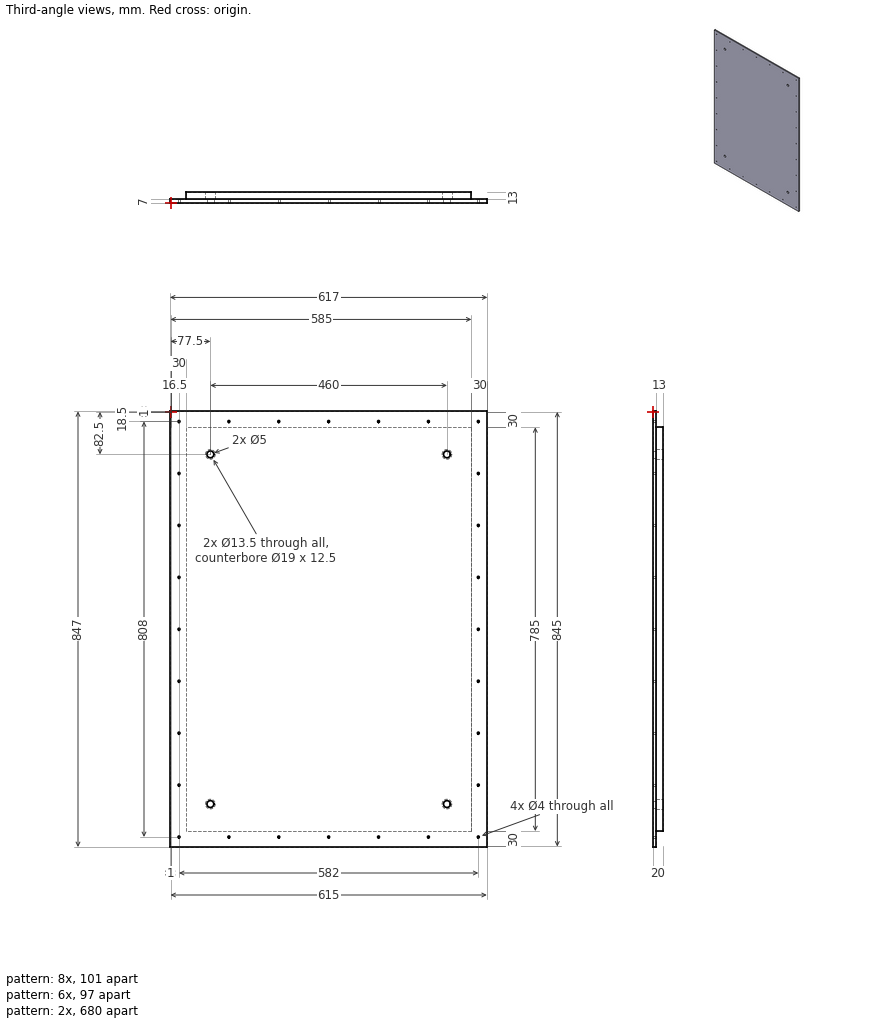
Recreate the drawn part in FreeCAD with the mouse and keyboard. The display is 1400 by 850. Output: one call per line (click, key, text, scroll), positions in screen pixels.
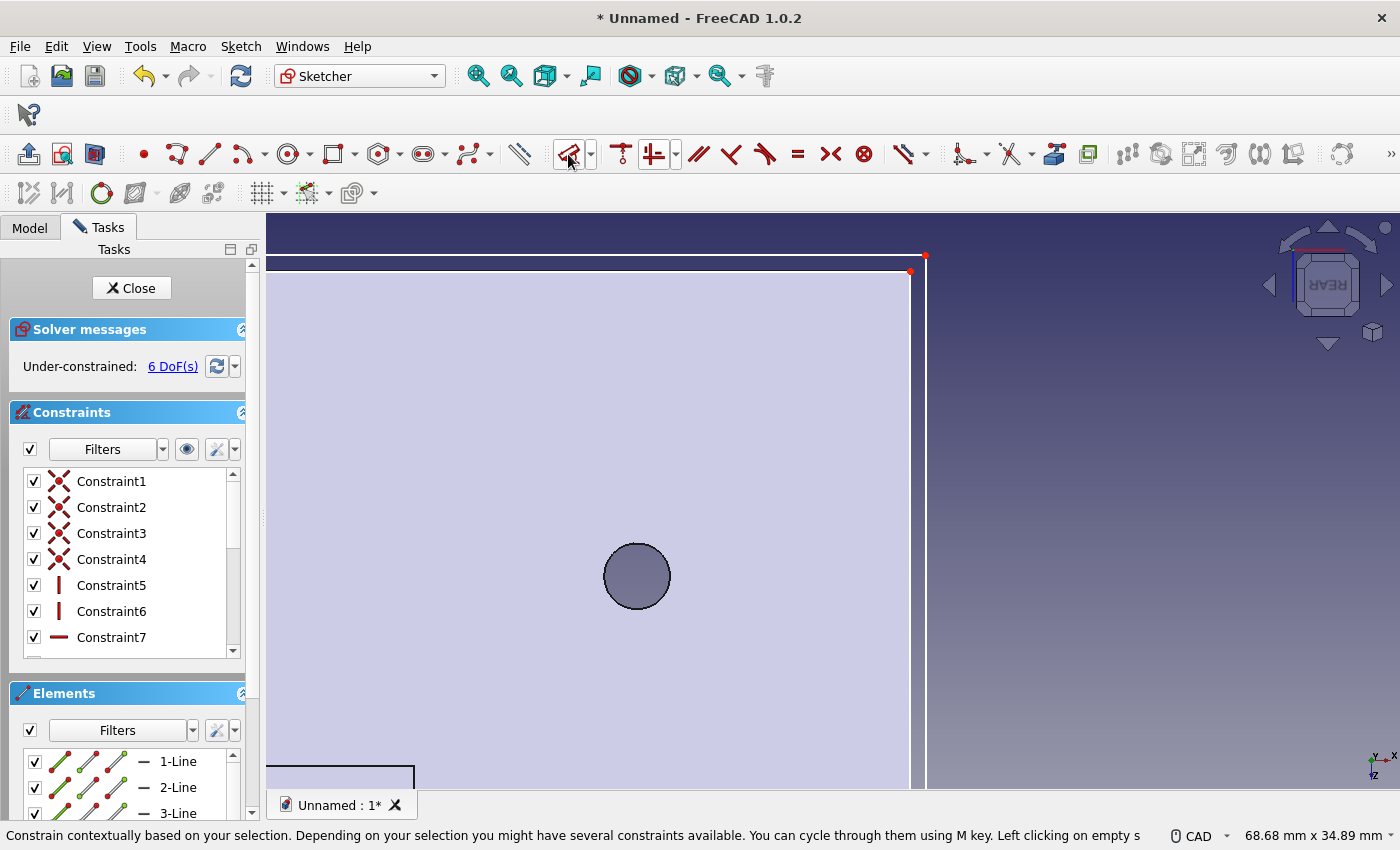
scroll(935, 268, down, 17)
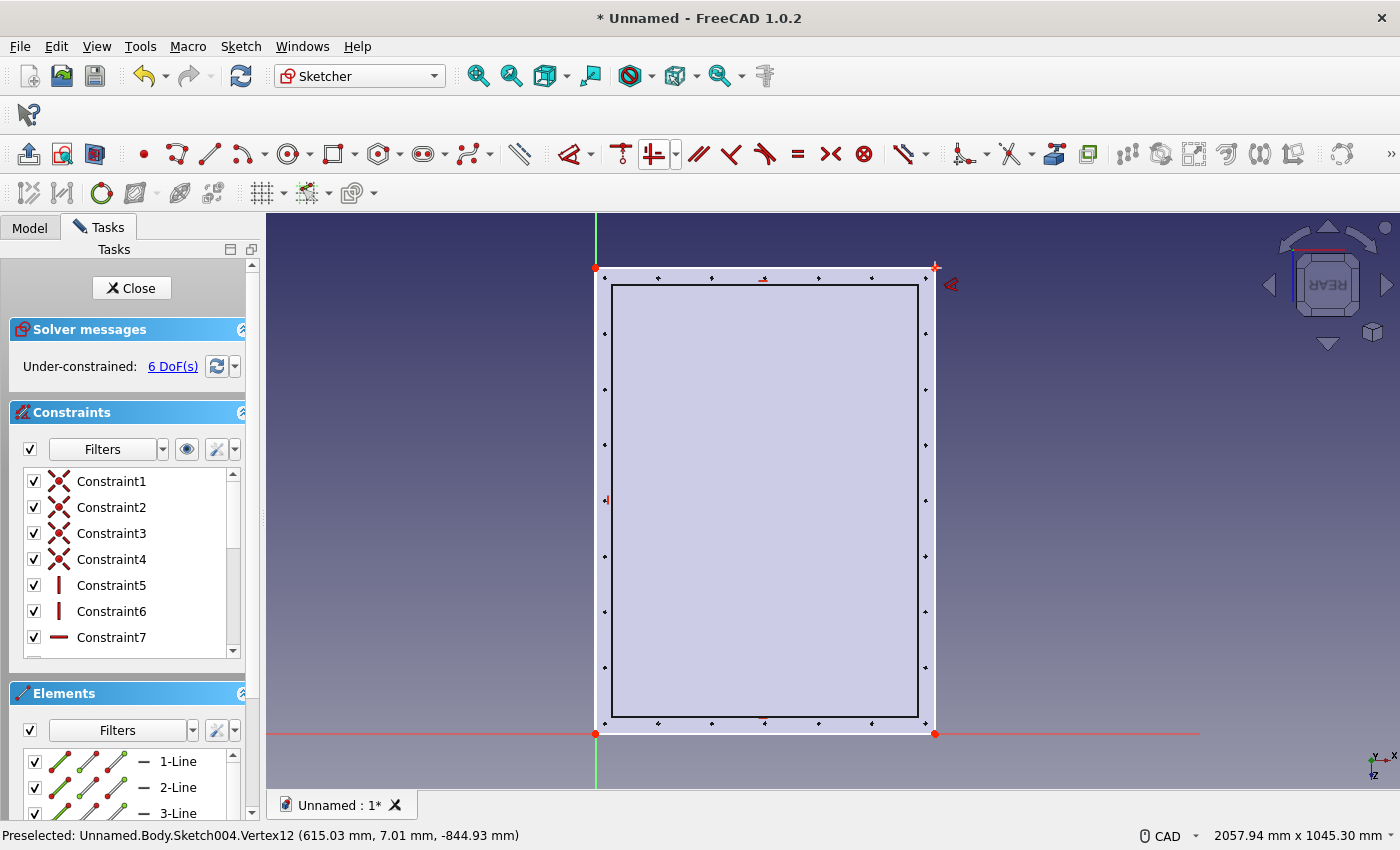
scroll(595, 268, up, 22)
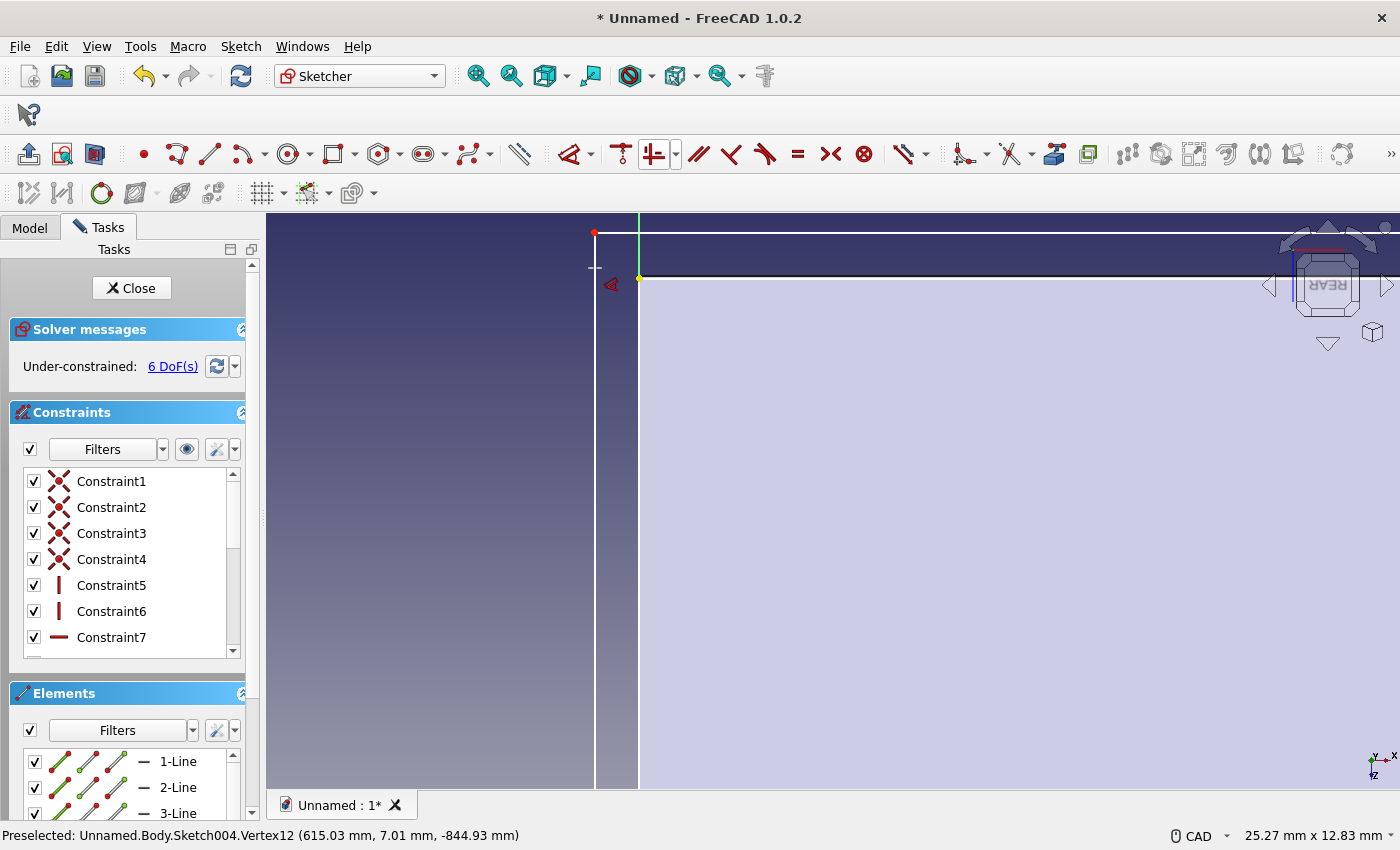
click(595, 233)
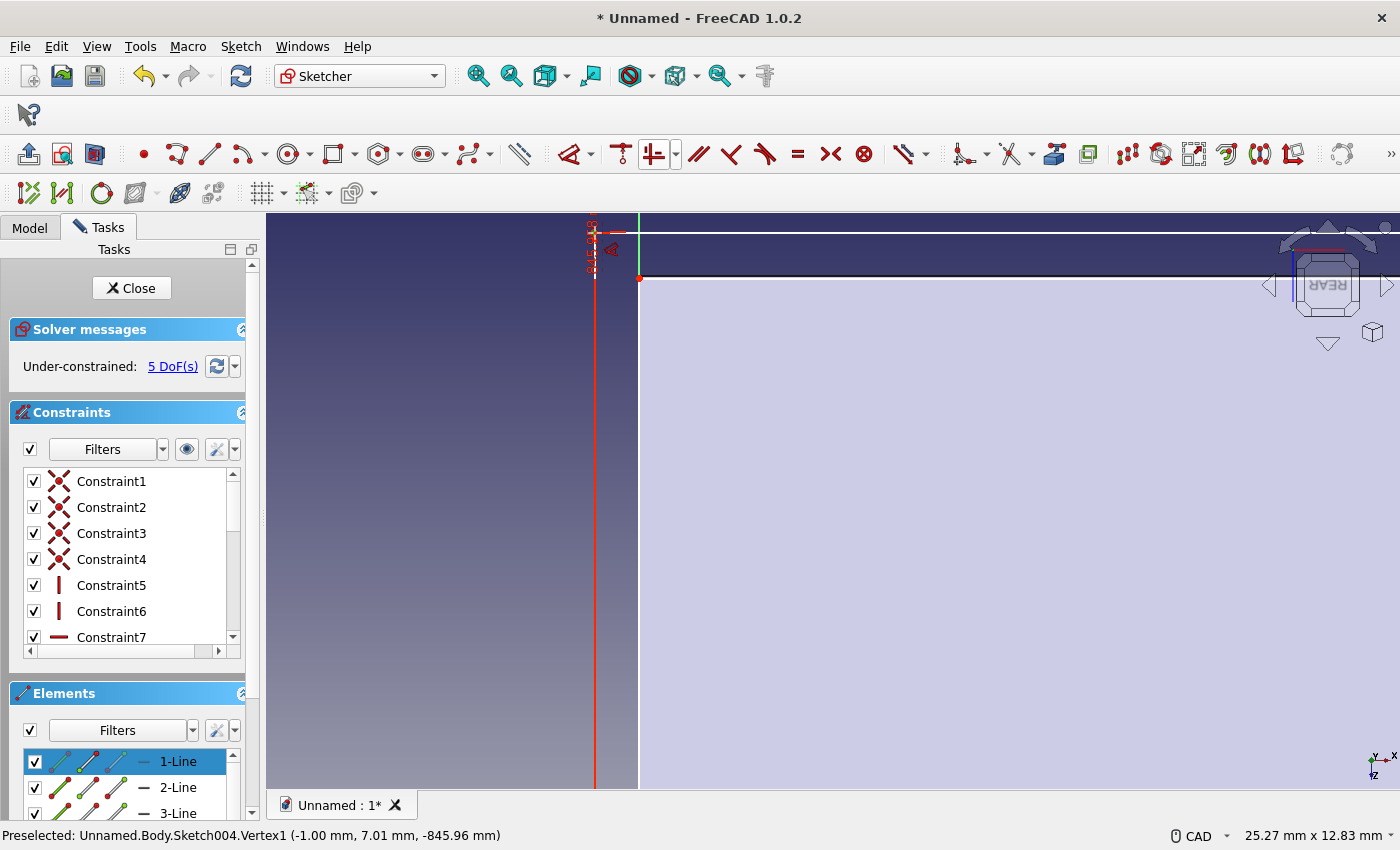
key(Escape)
key(Escape)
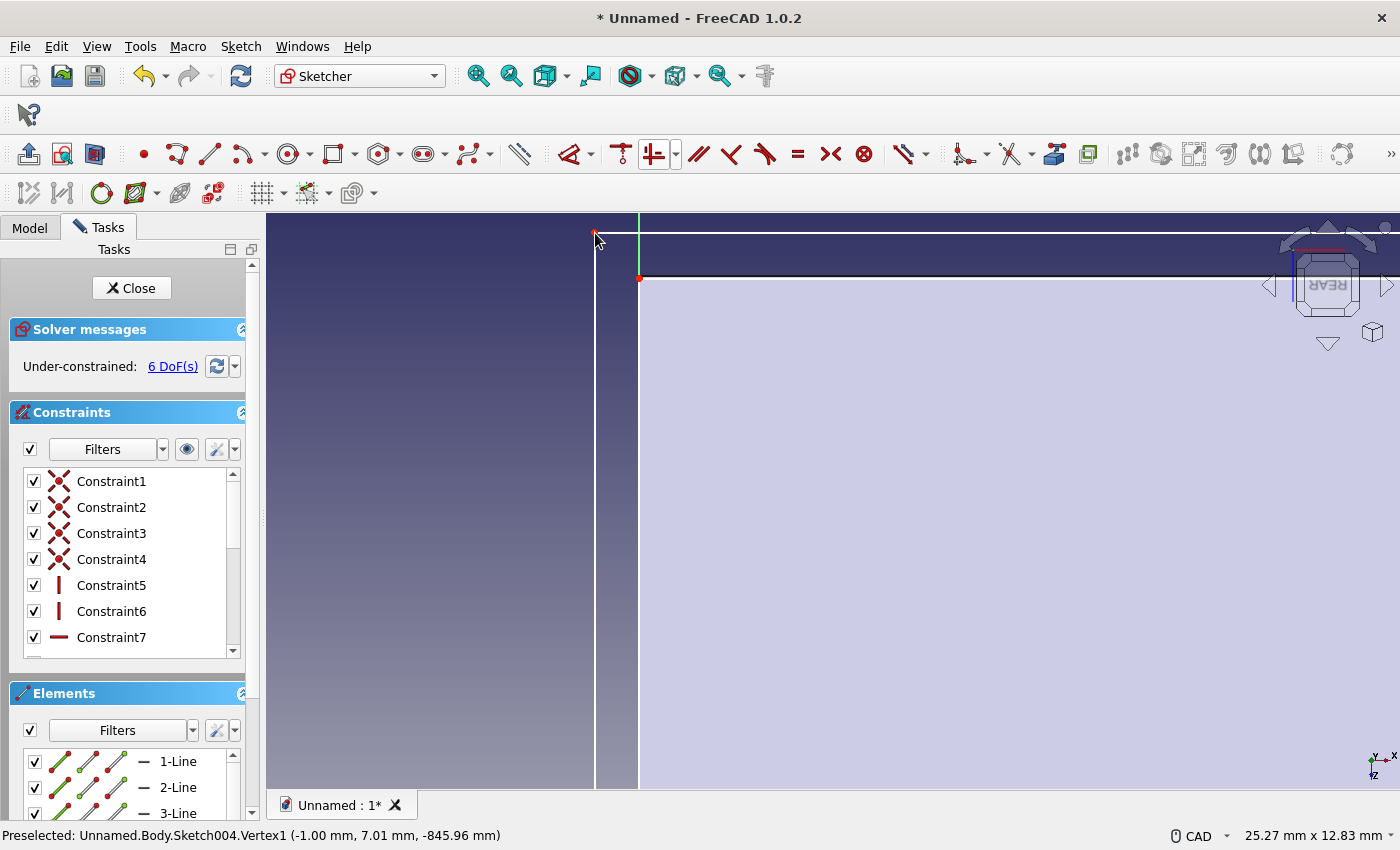
scroll(764, 501, down, 15)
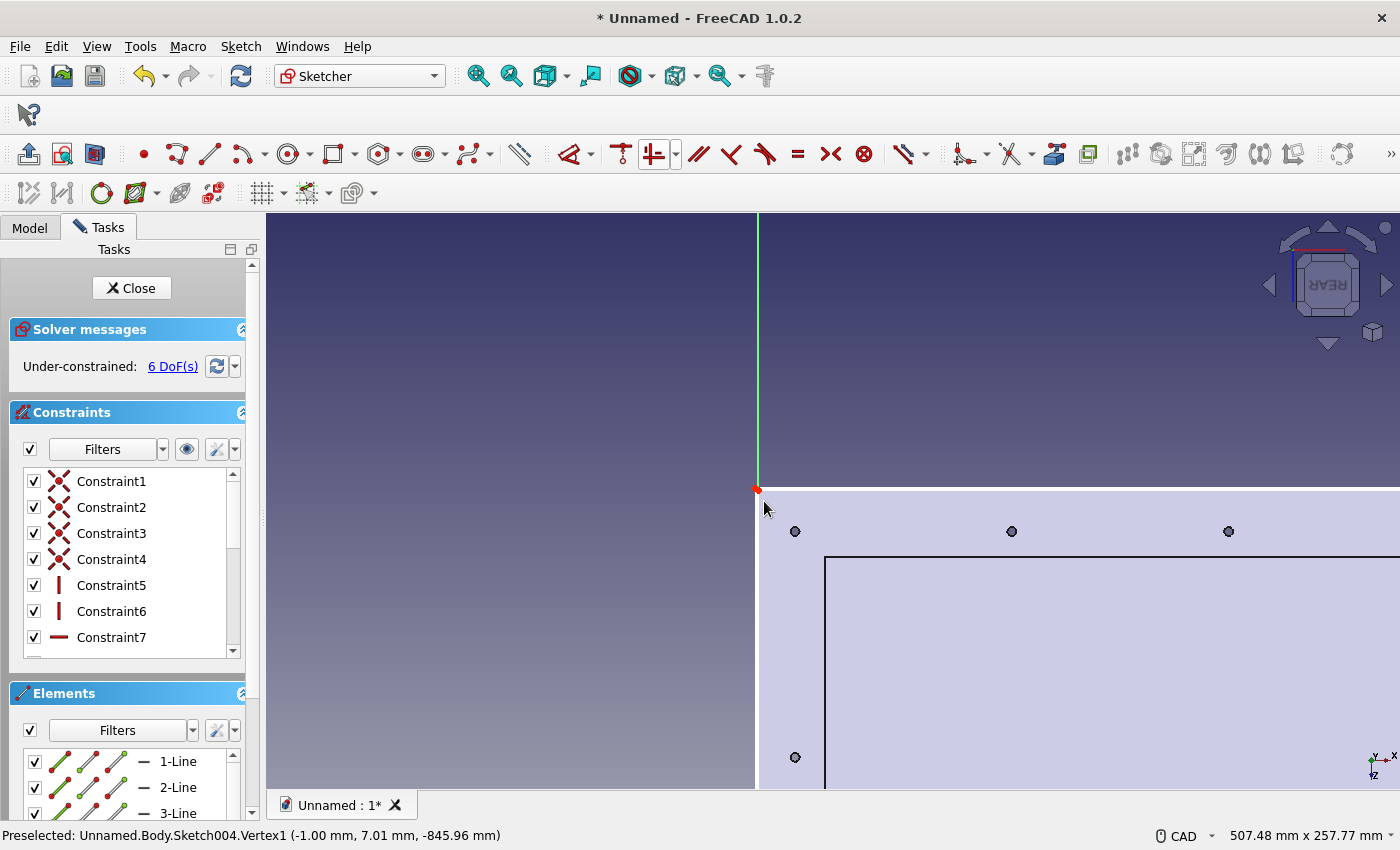
scroll(592, 265, down, 8)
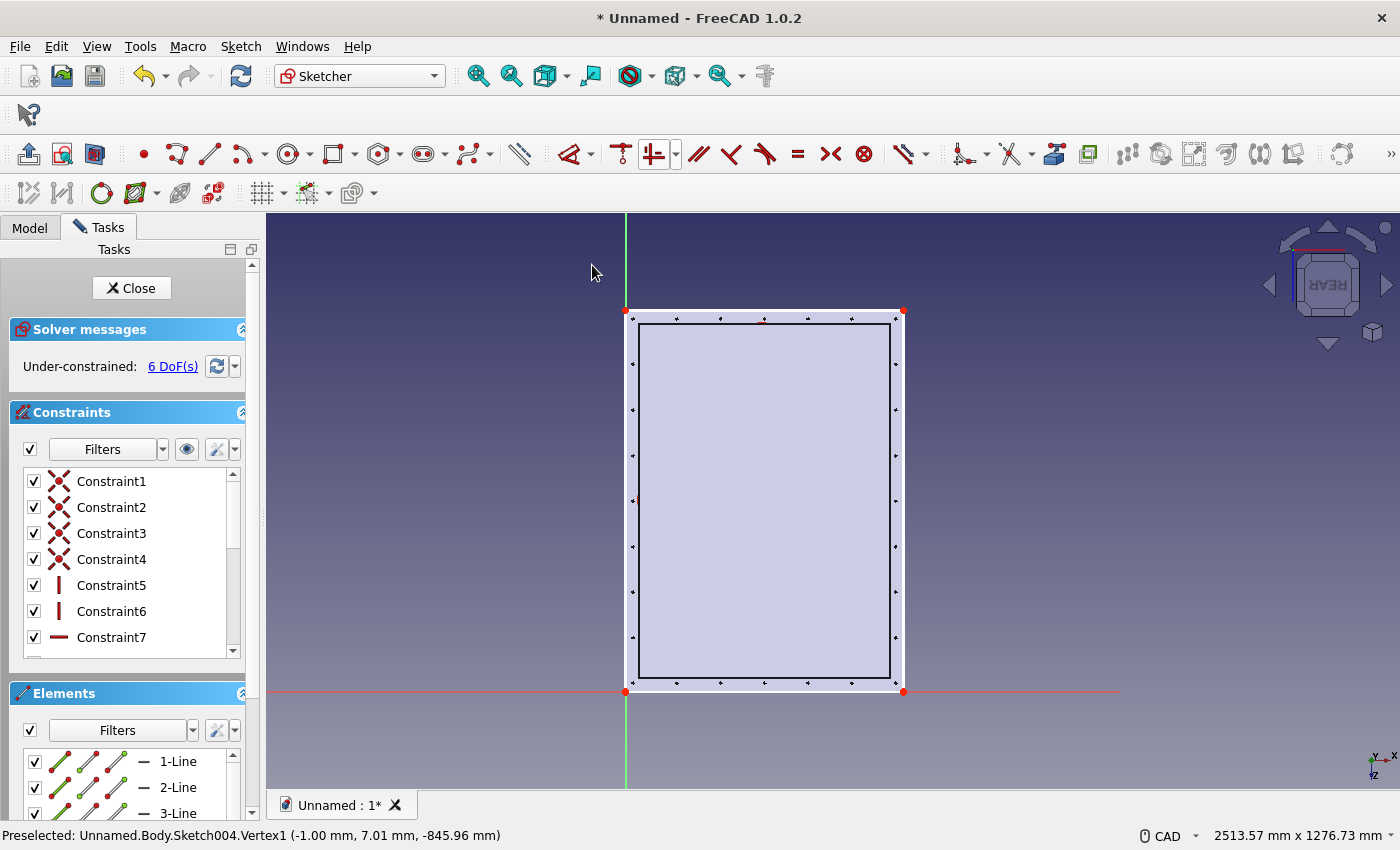
scroll(625, 310, up, 23)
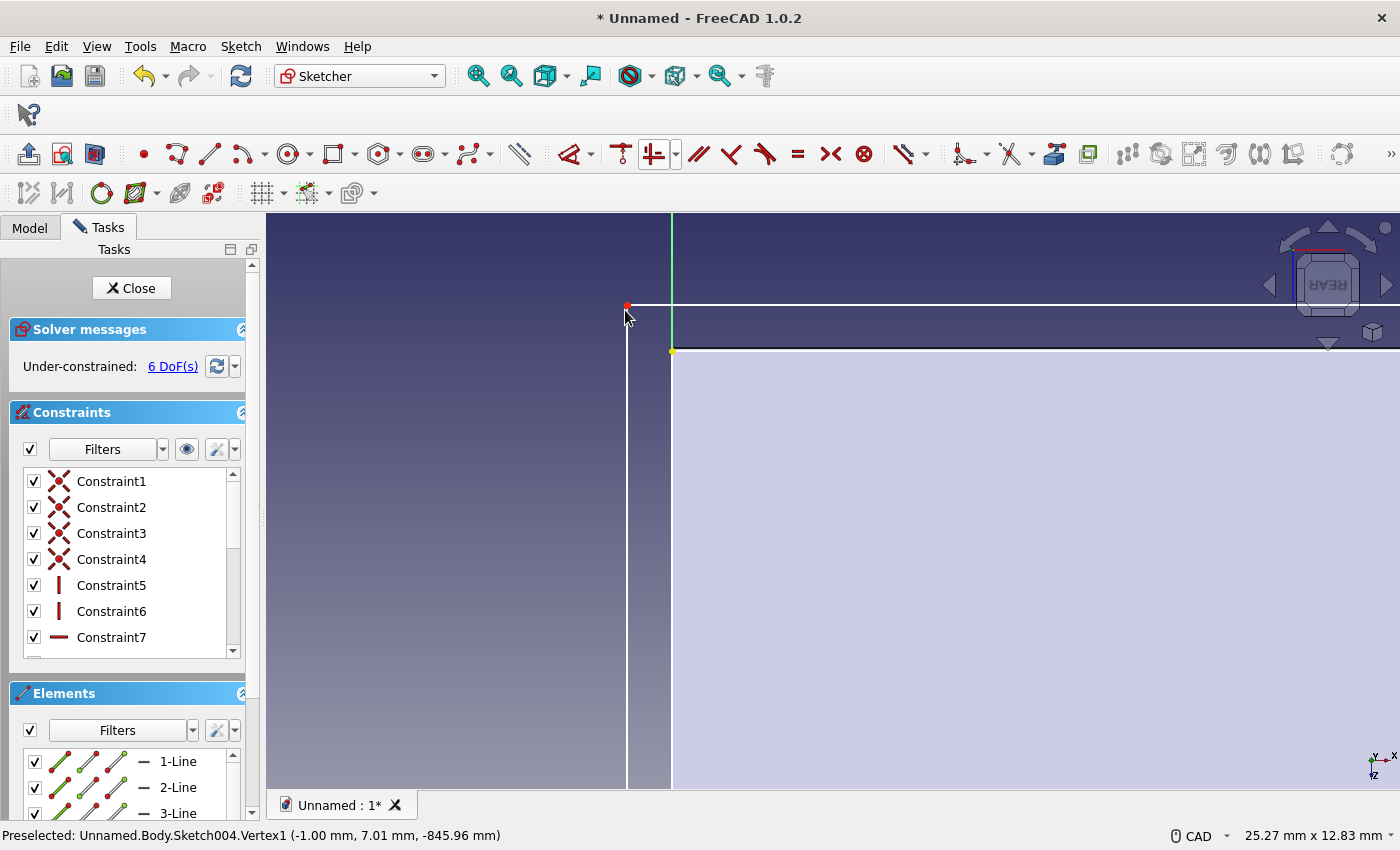
click(627, 305)